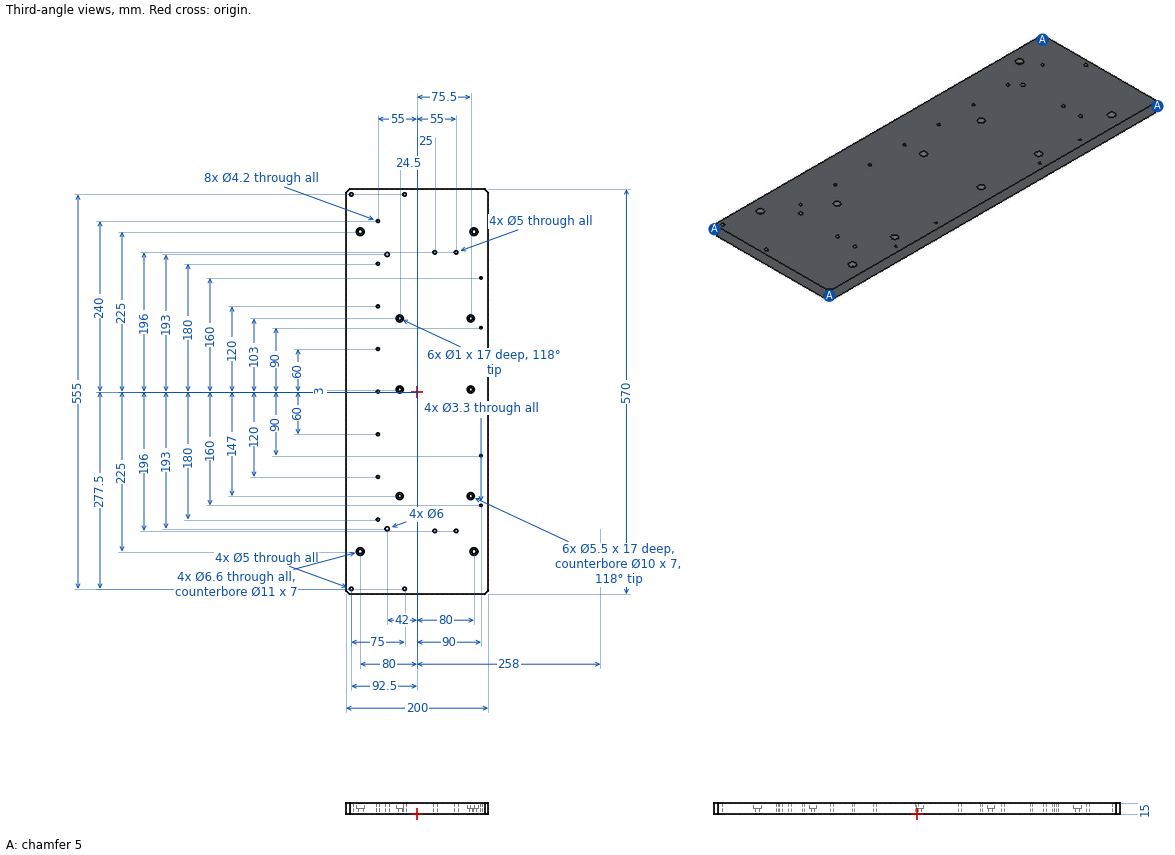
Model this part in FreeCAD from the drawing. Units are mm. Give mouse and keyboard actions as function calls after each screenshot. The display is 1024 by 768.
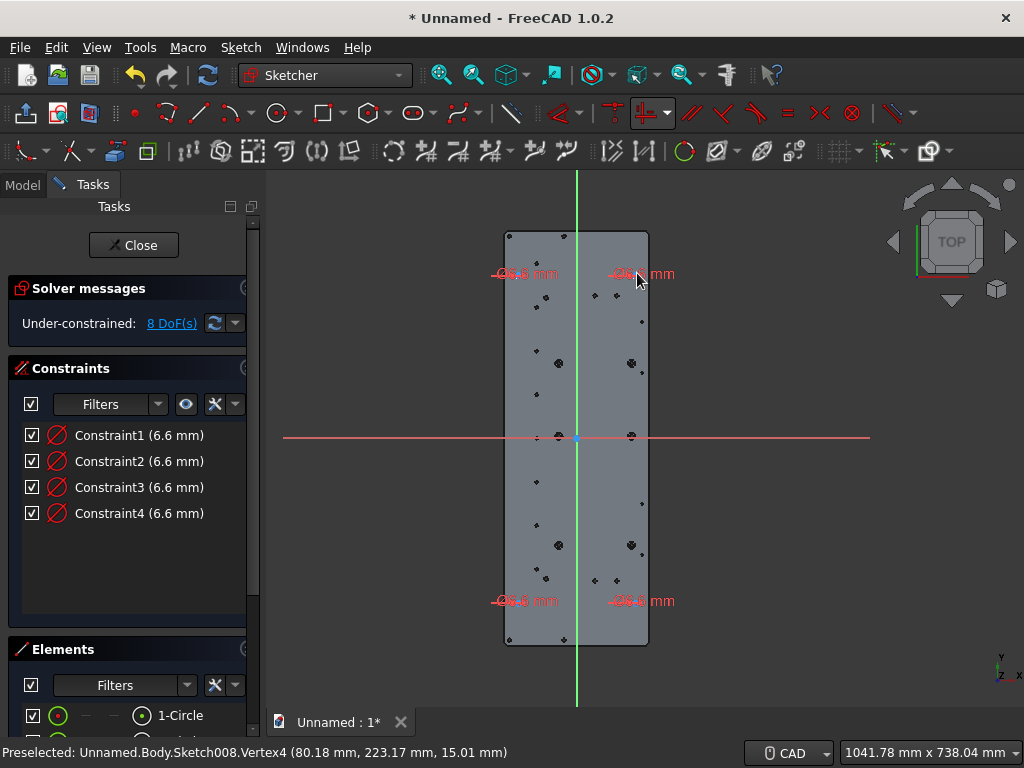
click(518, 603)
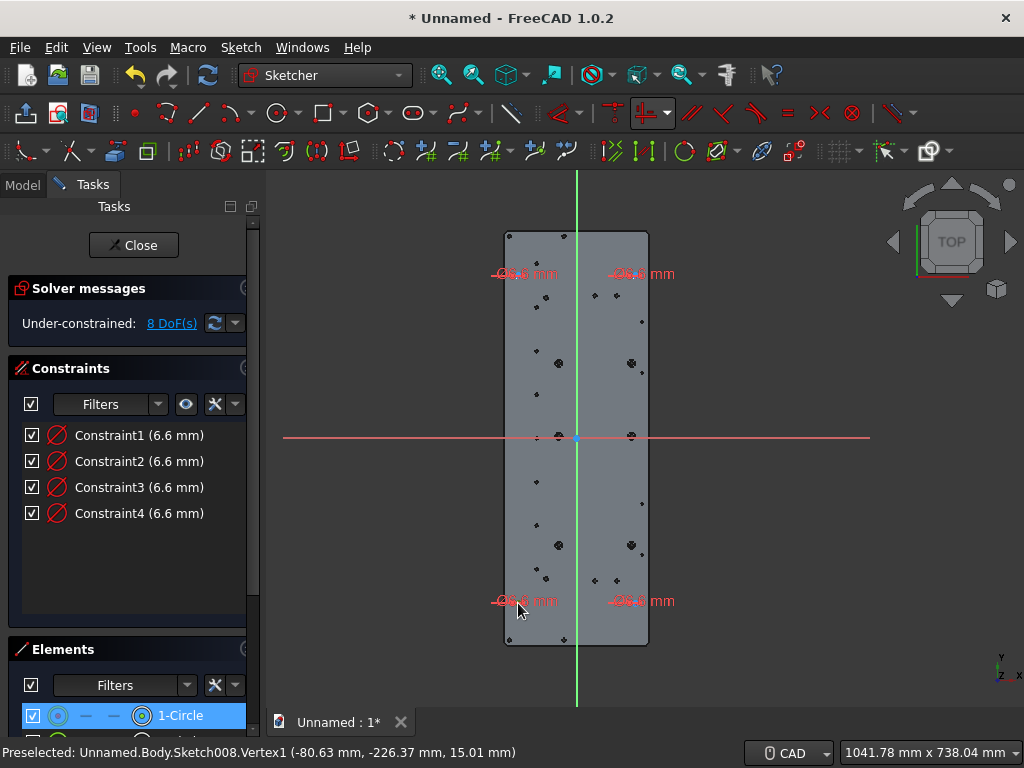
click(635, 603)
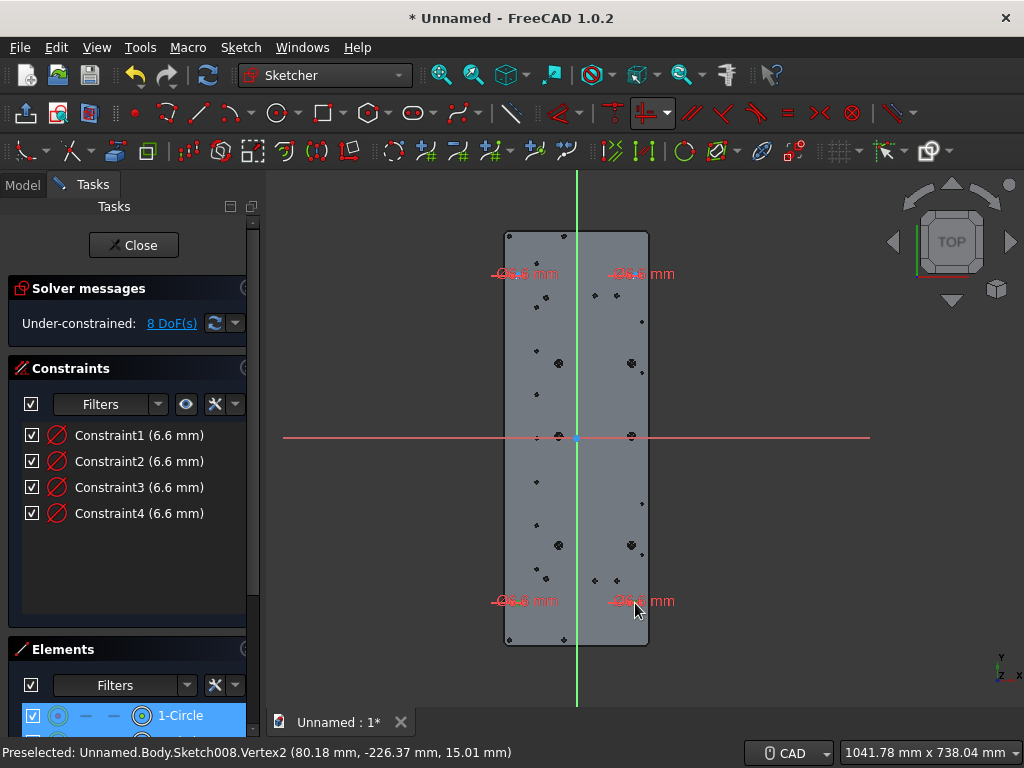
click(670, 114)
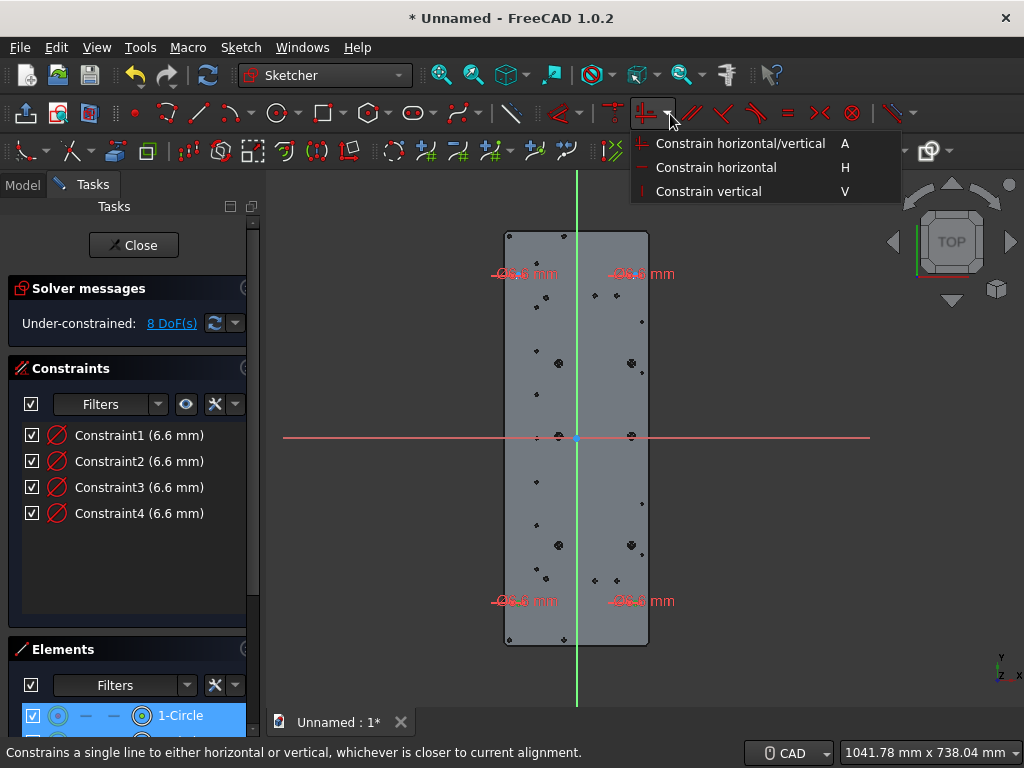
click(766, 167)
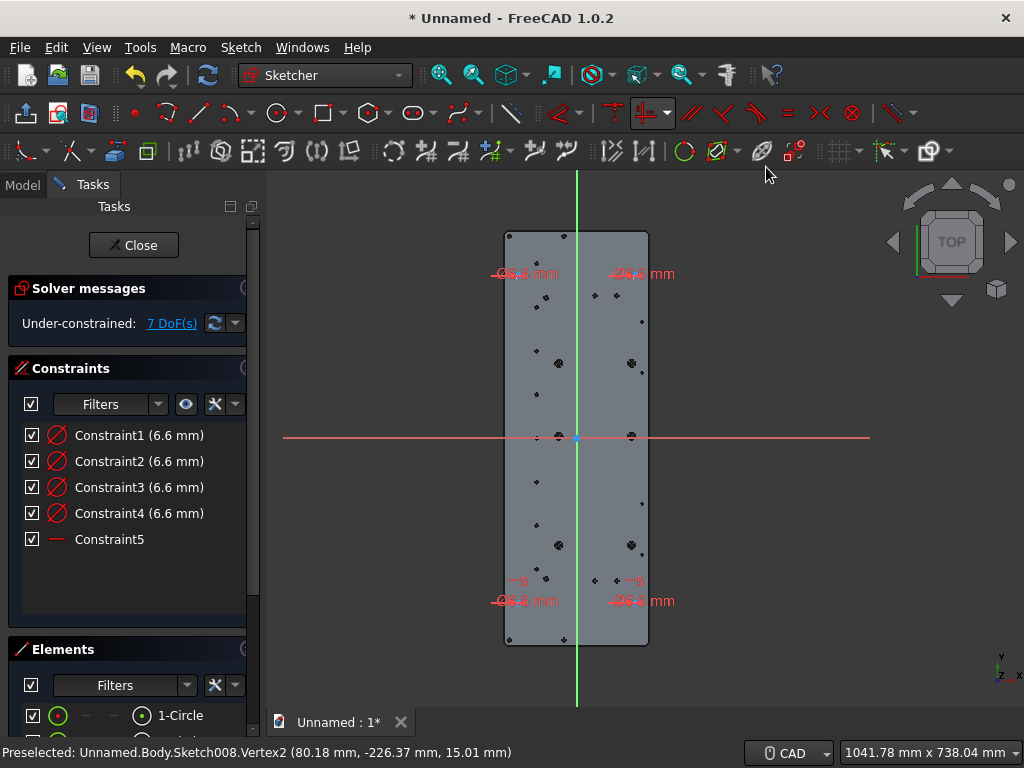
click(518, 603)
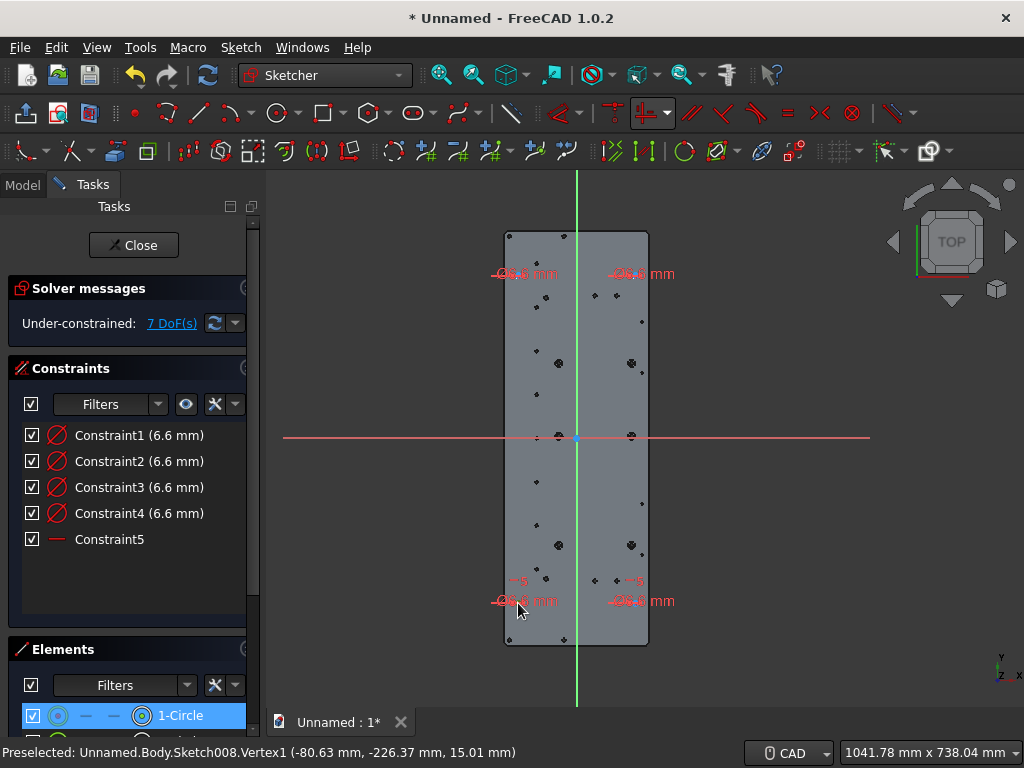
click(518, 276)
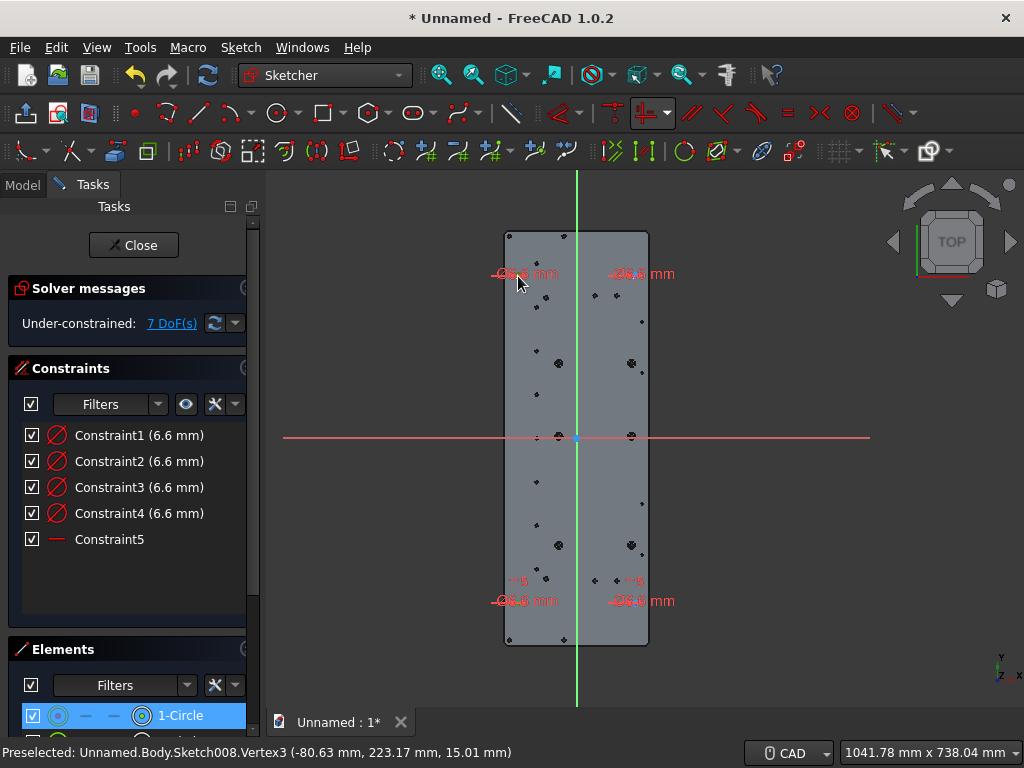
click(670, 114)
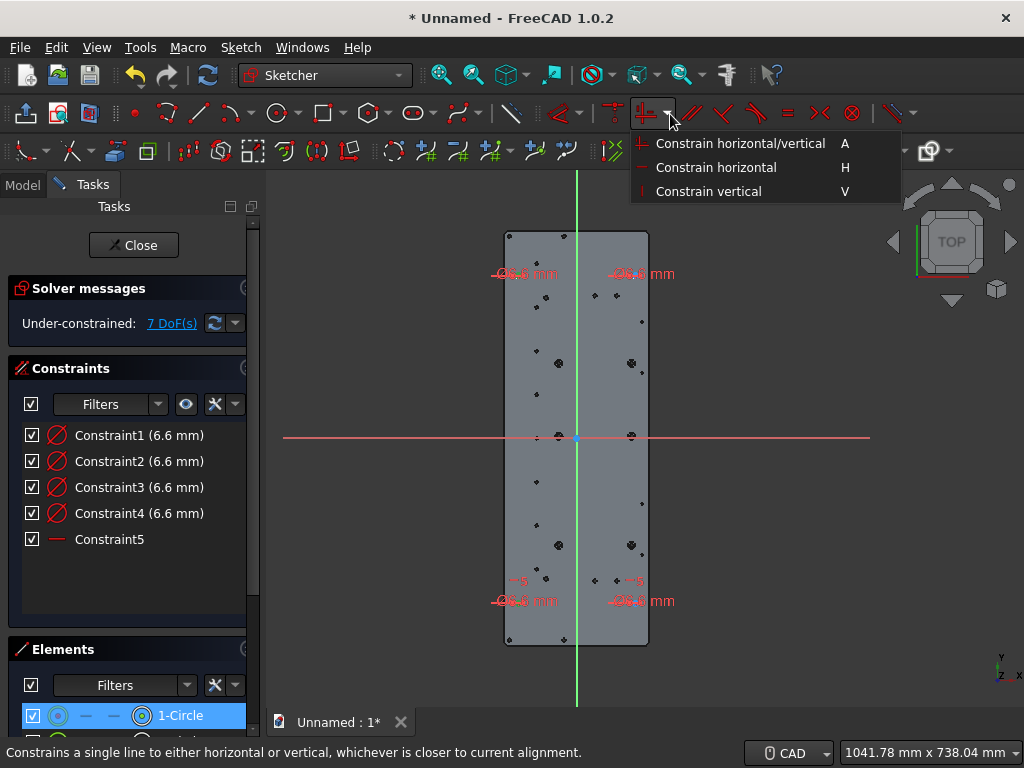
click(766, 191)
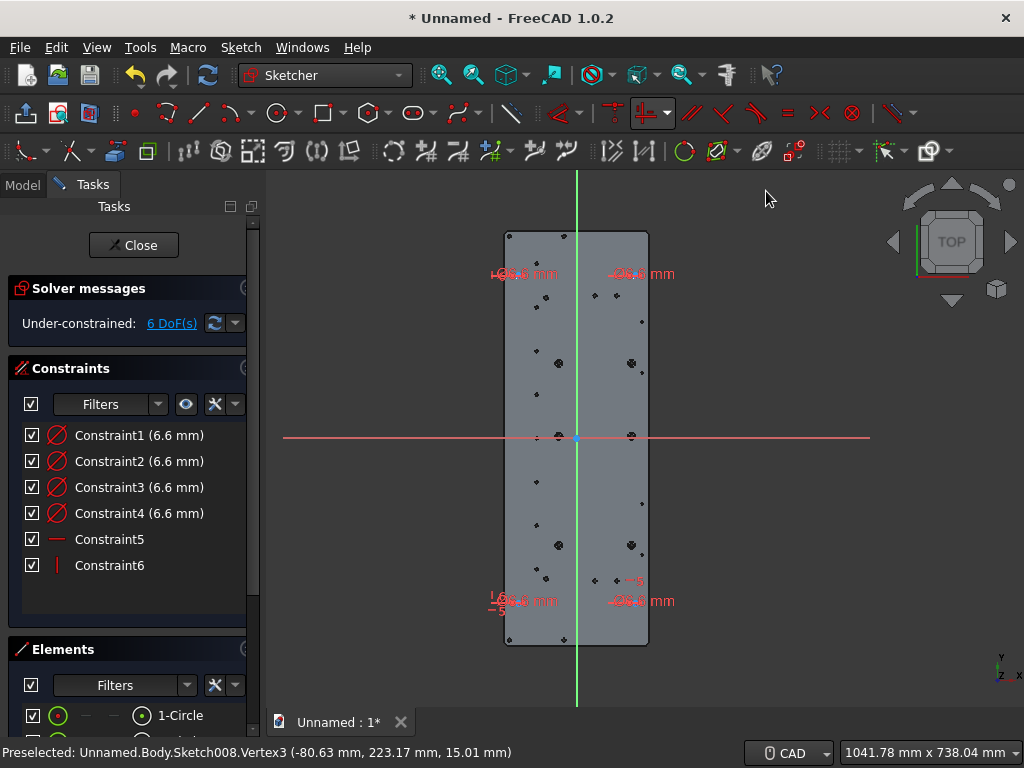
click(635, 603)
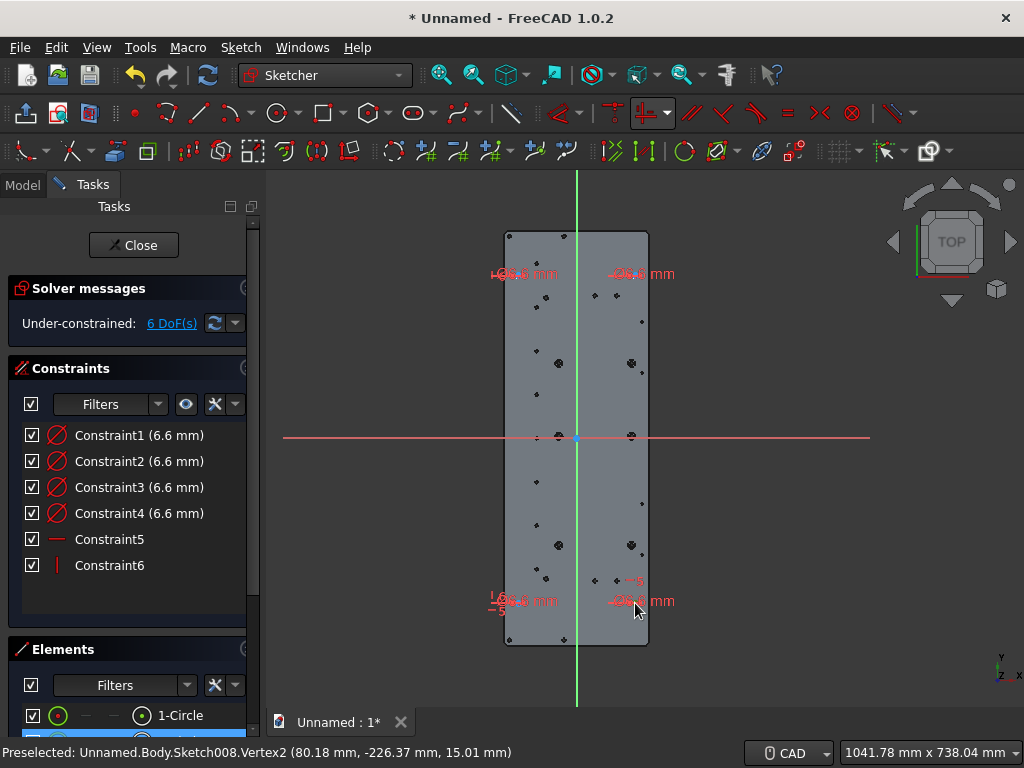
click(635, 276)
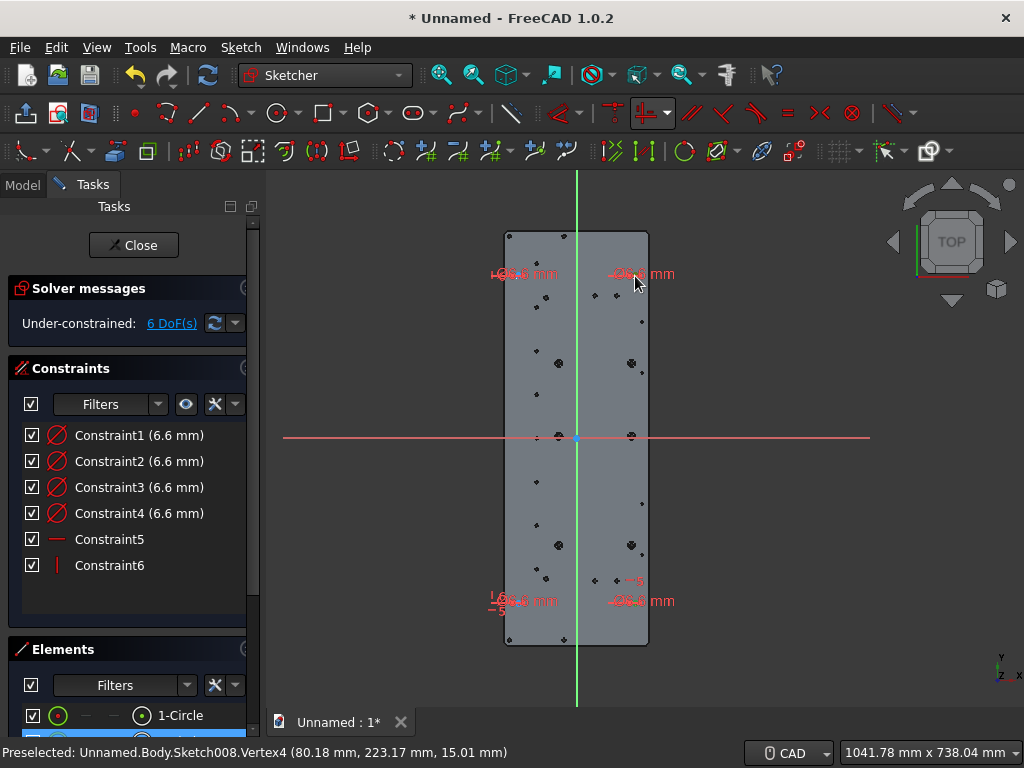
key(v)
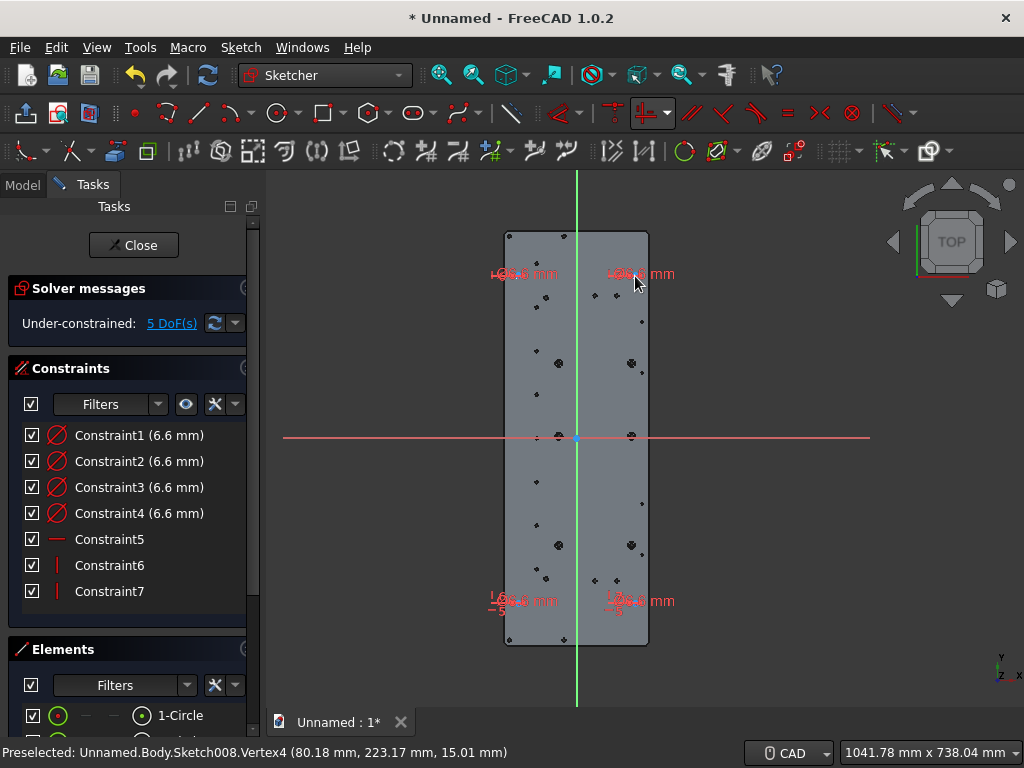
click(518, 276)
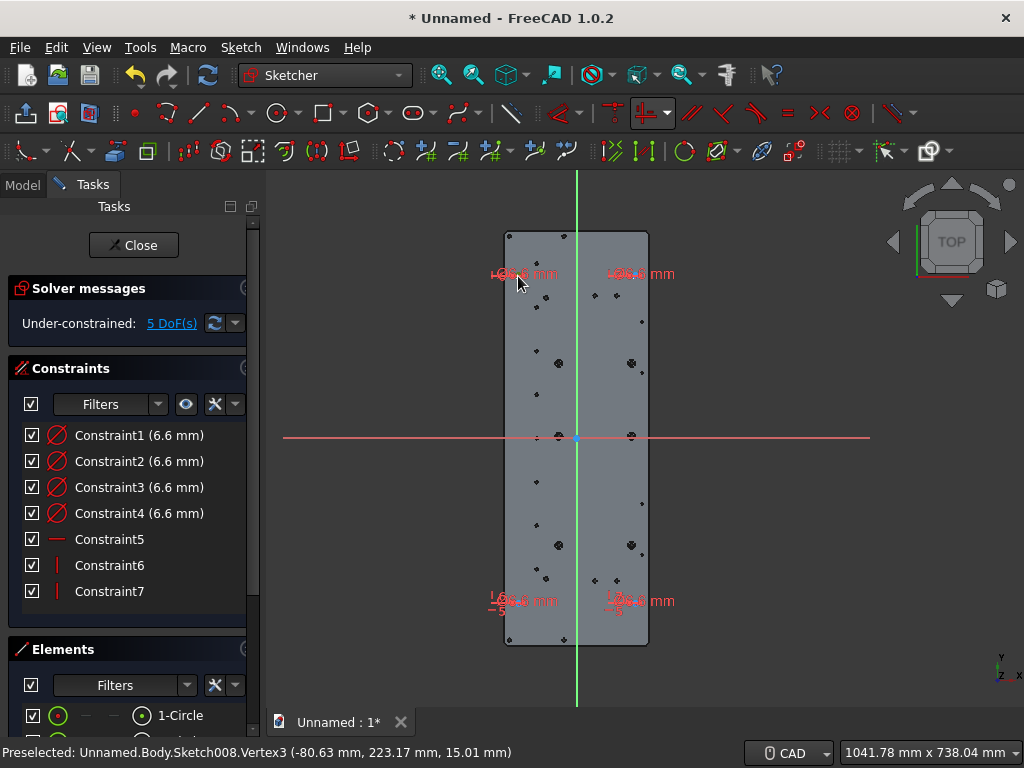
click(635, 276)